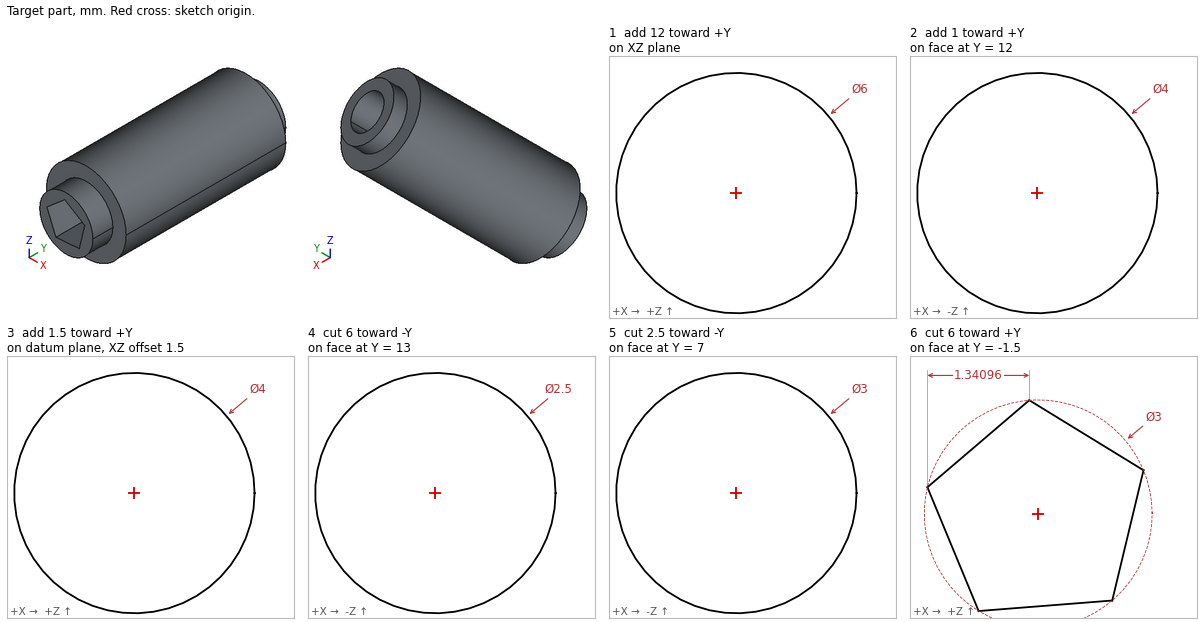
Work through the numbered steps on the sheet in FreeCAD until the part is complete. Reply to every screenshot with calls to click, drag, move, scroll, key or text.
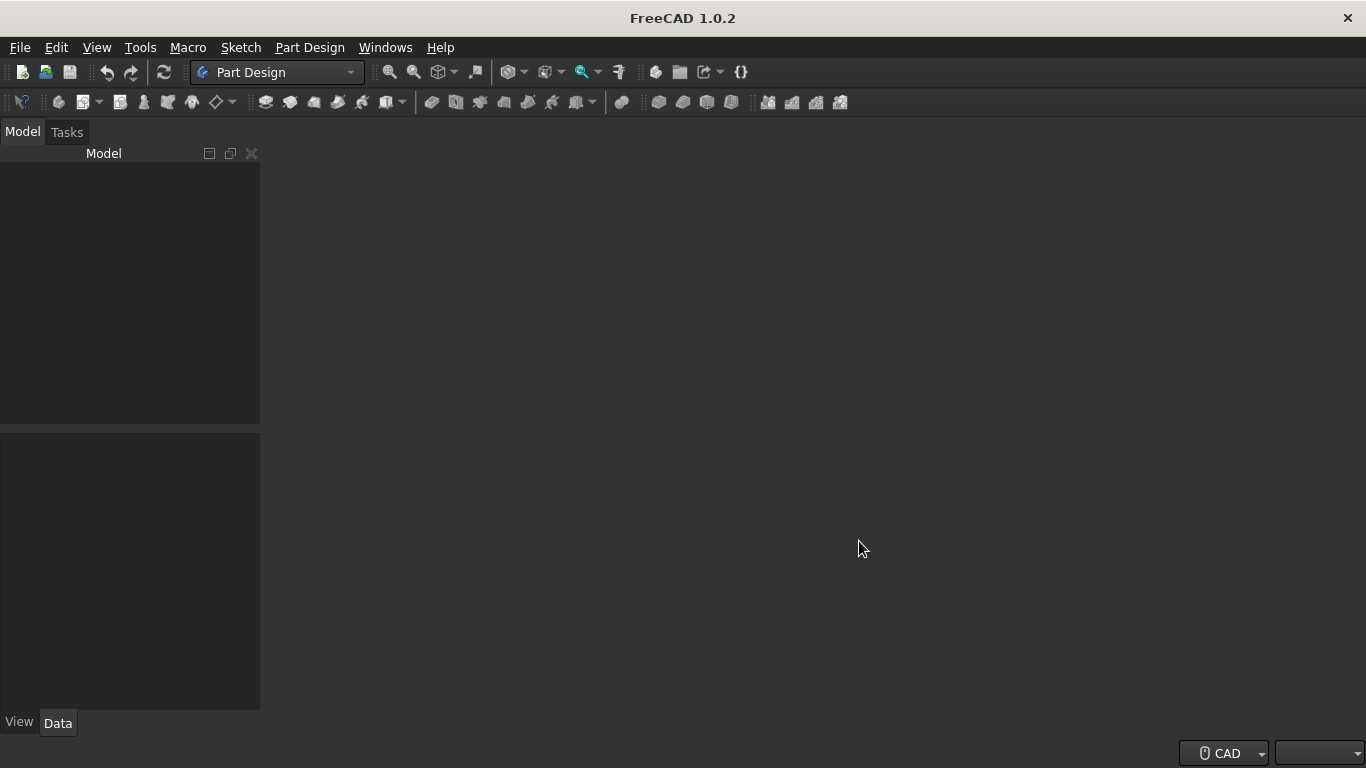
click(22, 72)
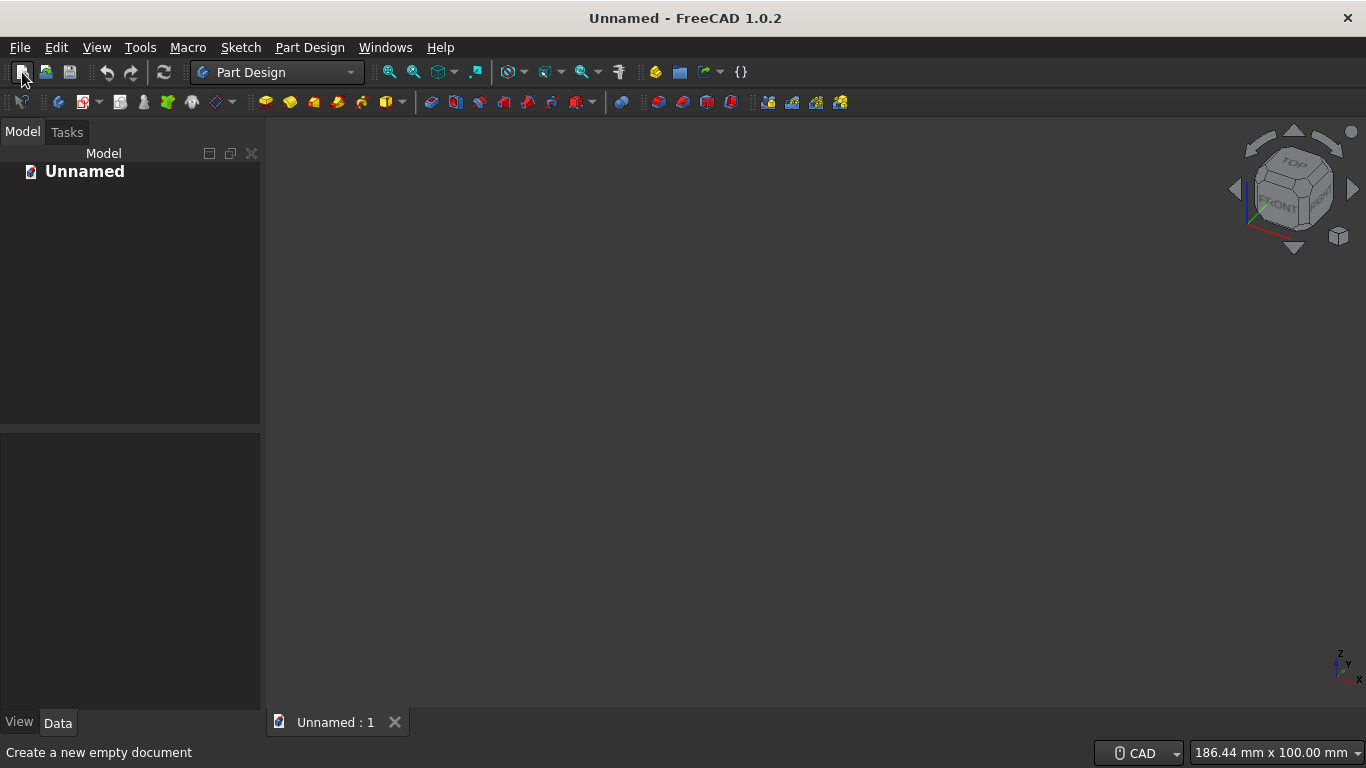
click(84, 102)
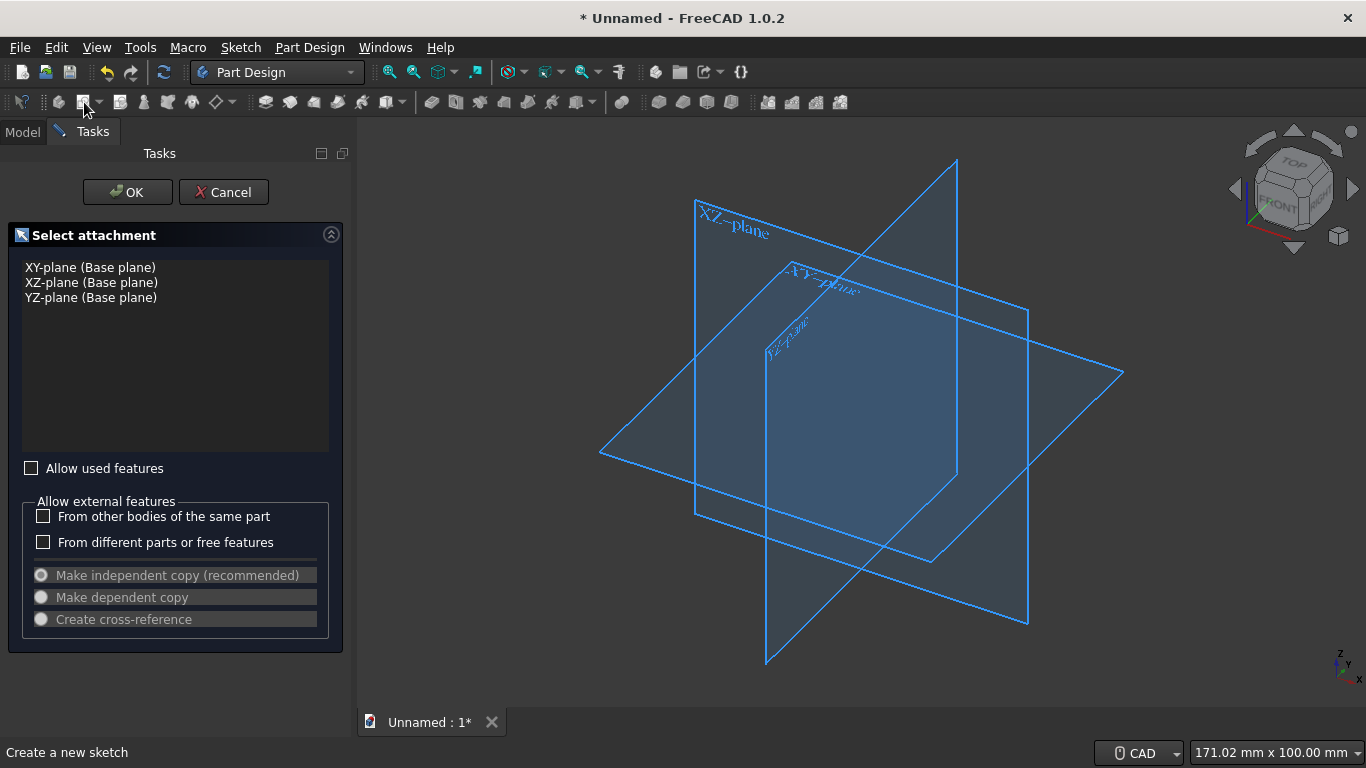
click(82, 282)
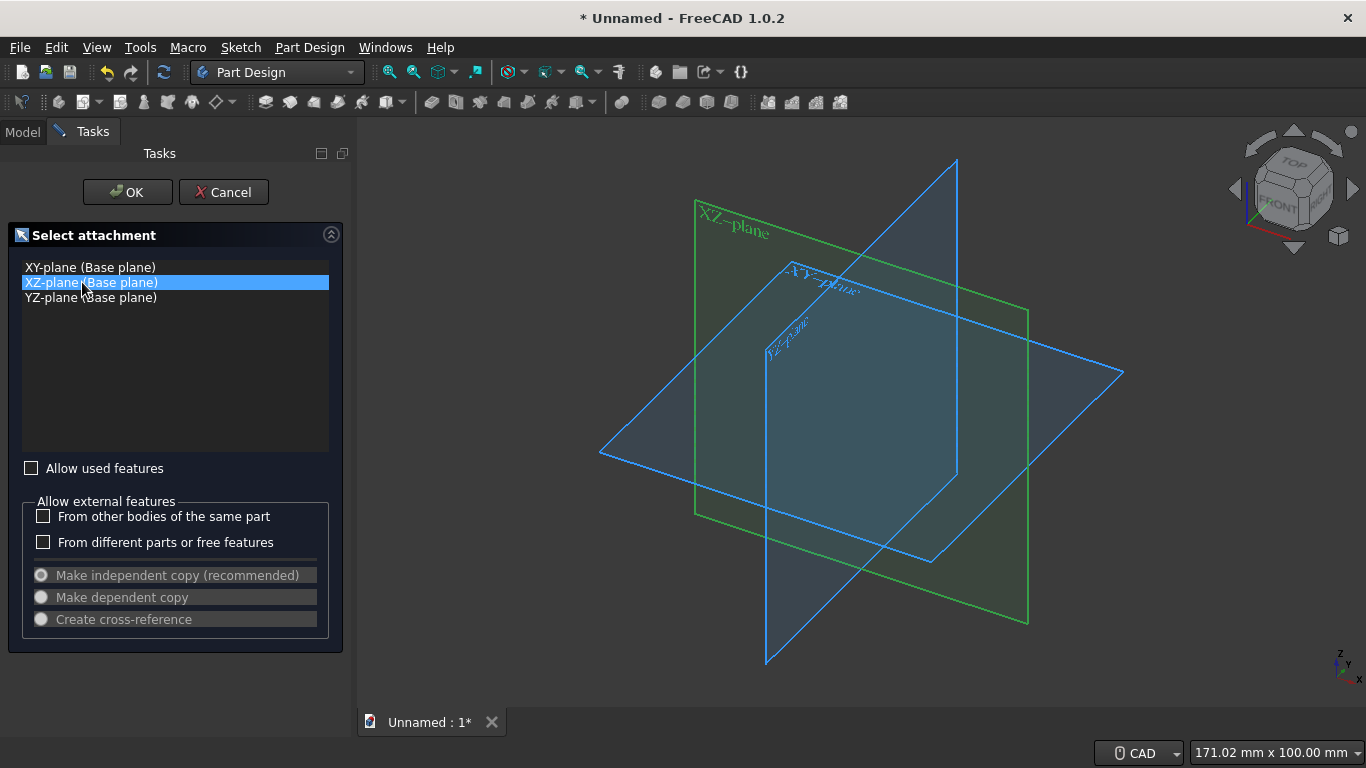
click(128, 192)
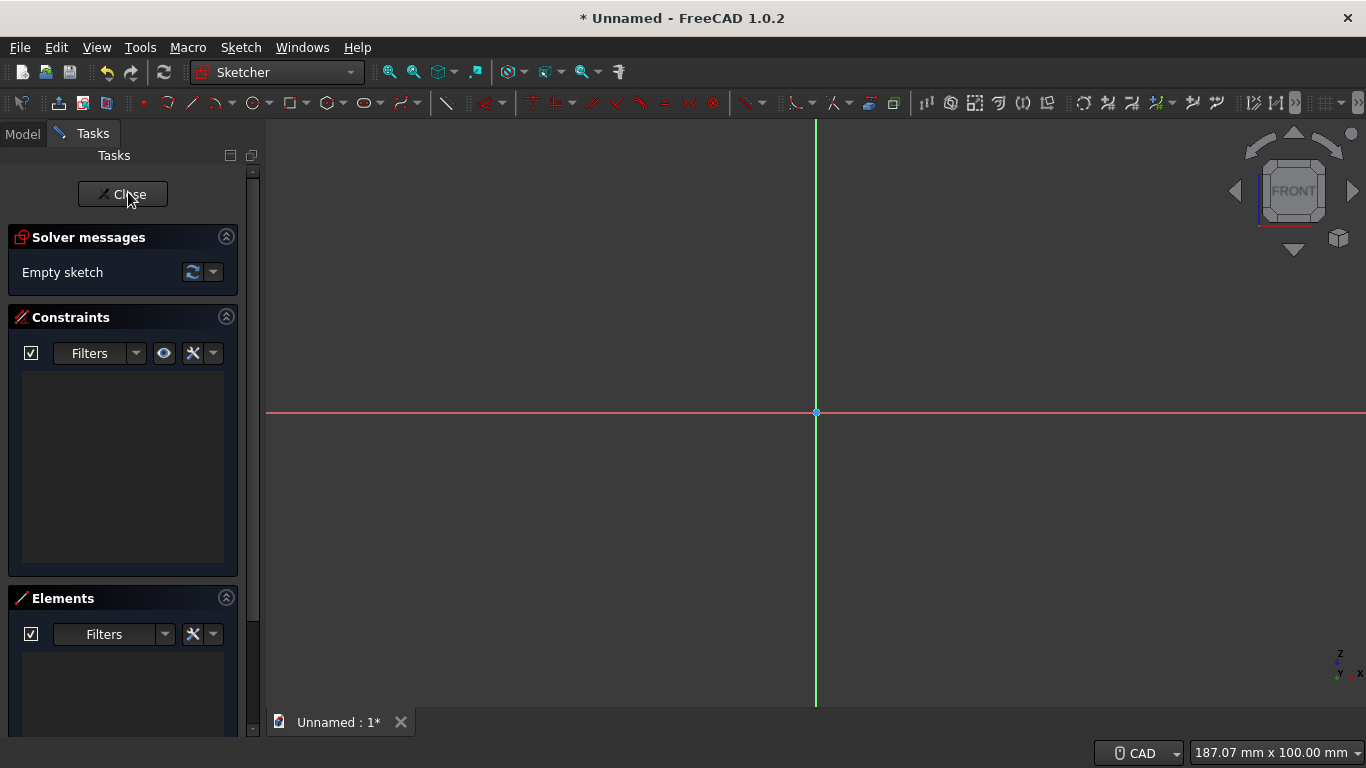
scroll(823, 413, up, 12)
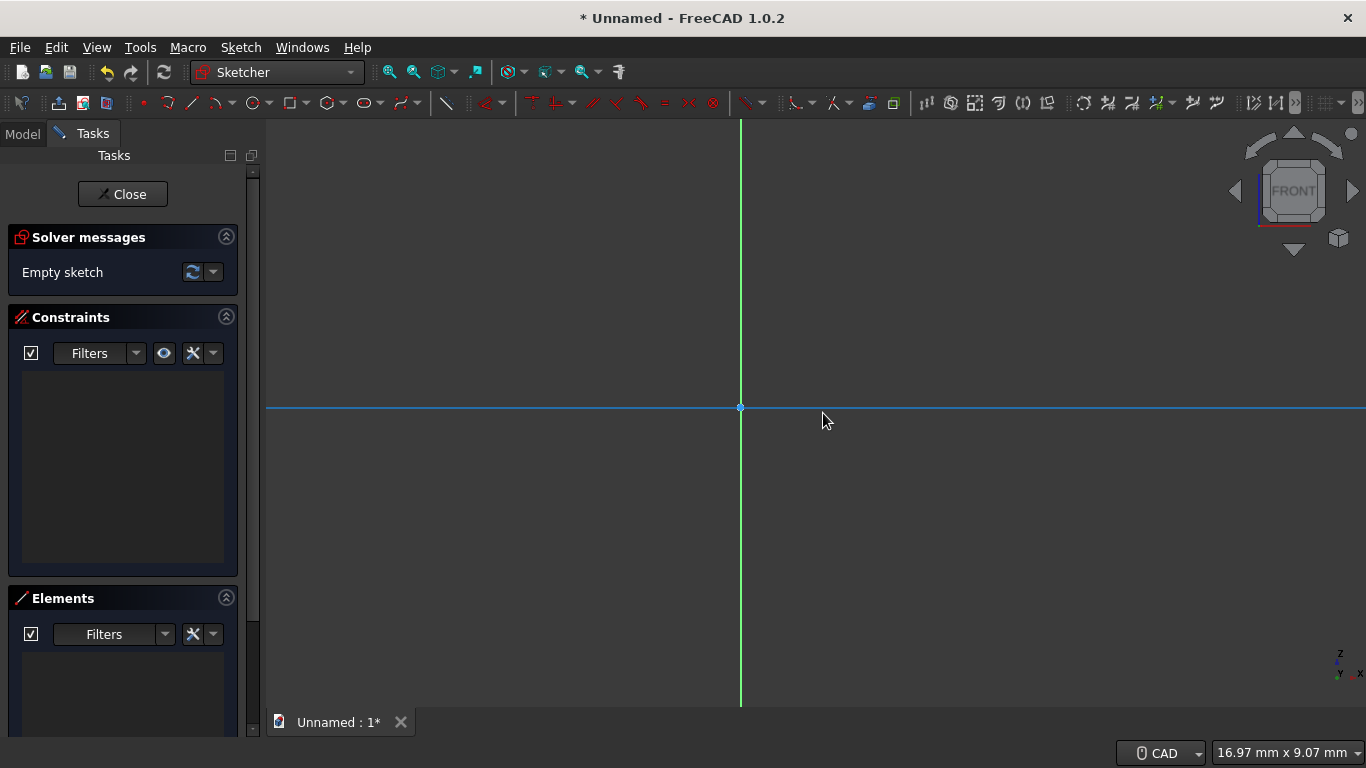
click(254, 104)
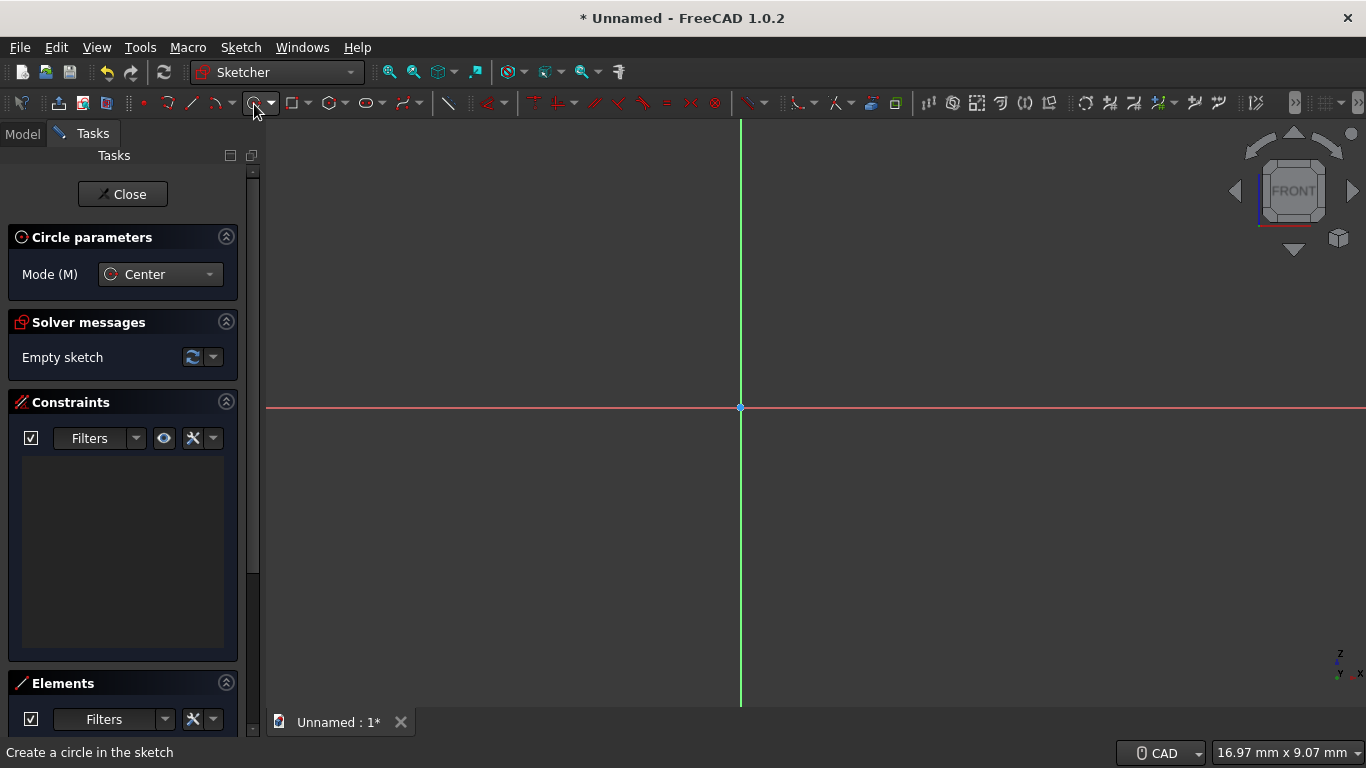
click(741, 408)
move(878, 270)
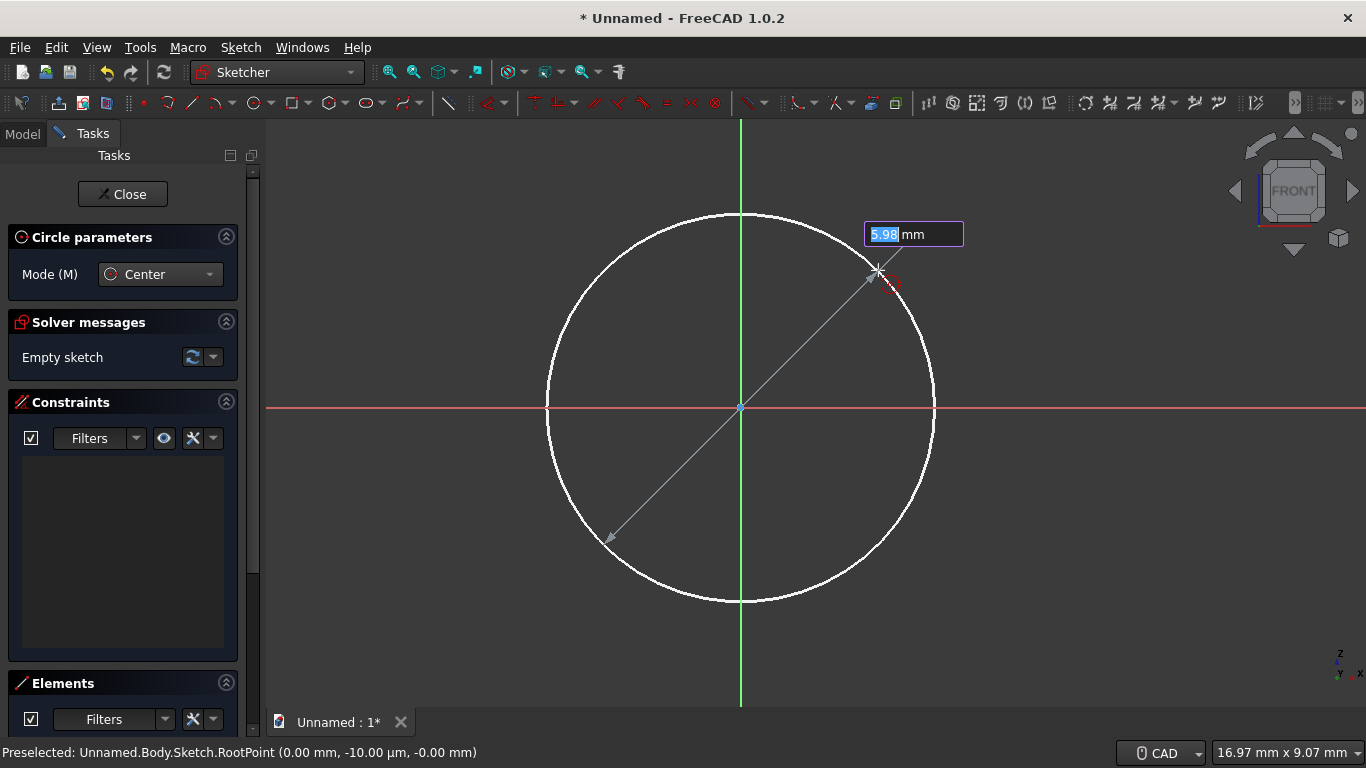
text(6)
key(Return)
key(Escape)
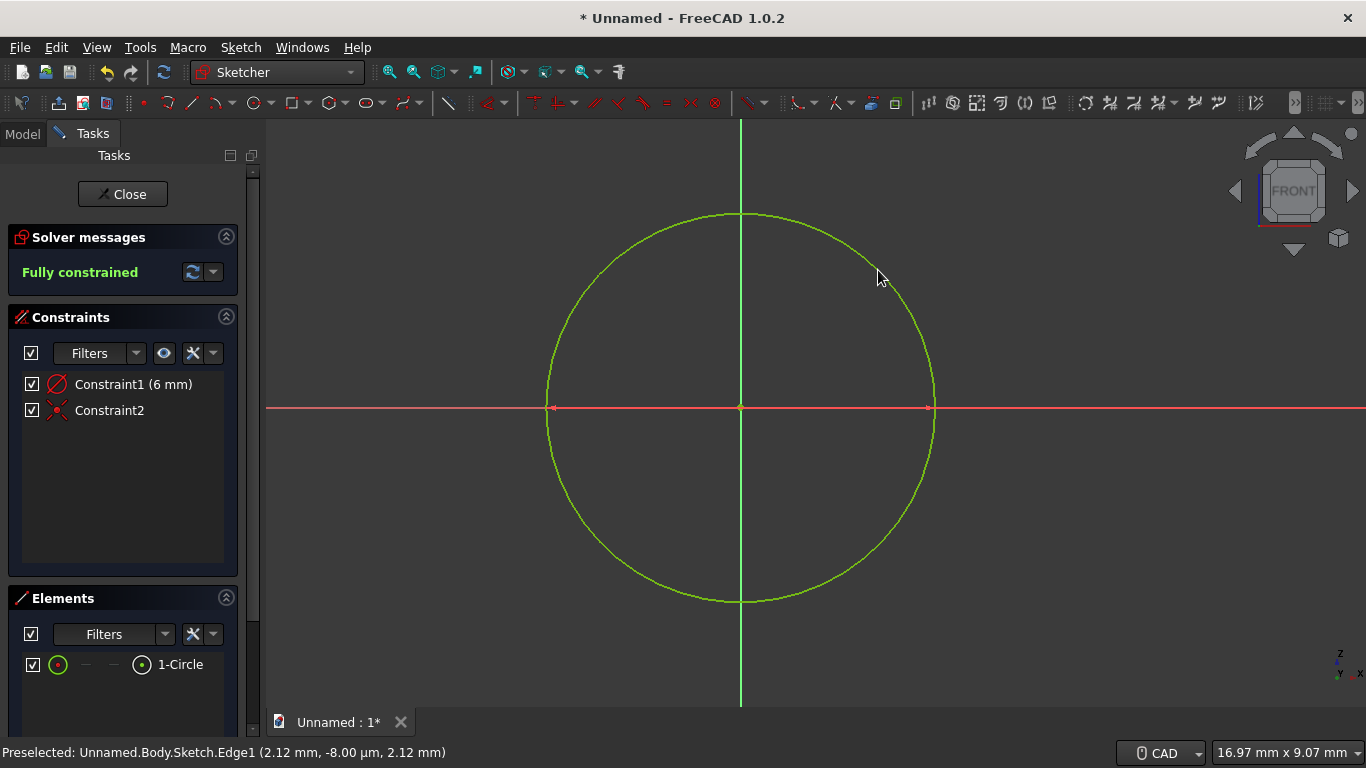
click(123, 194)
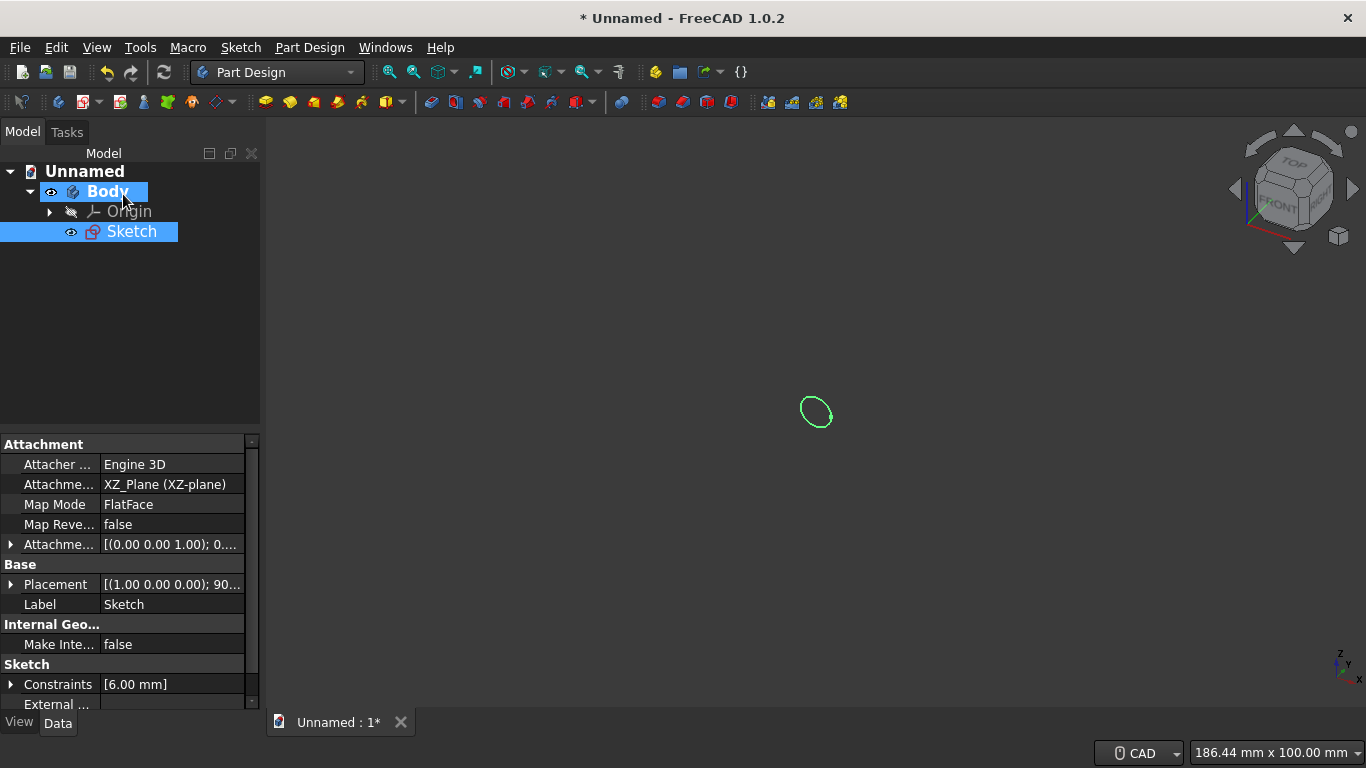
click(266, 102)